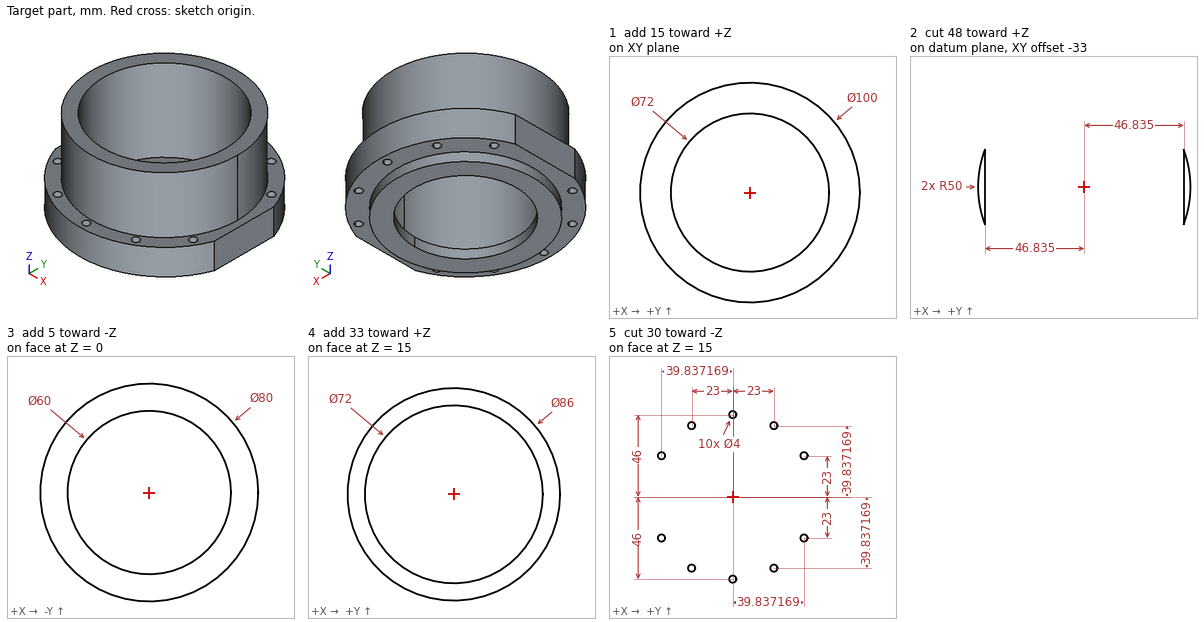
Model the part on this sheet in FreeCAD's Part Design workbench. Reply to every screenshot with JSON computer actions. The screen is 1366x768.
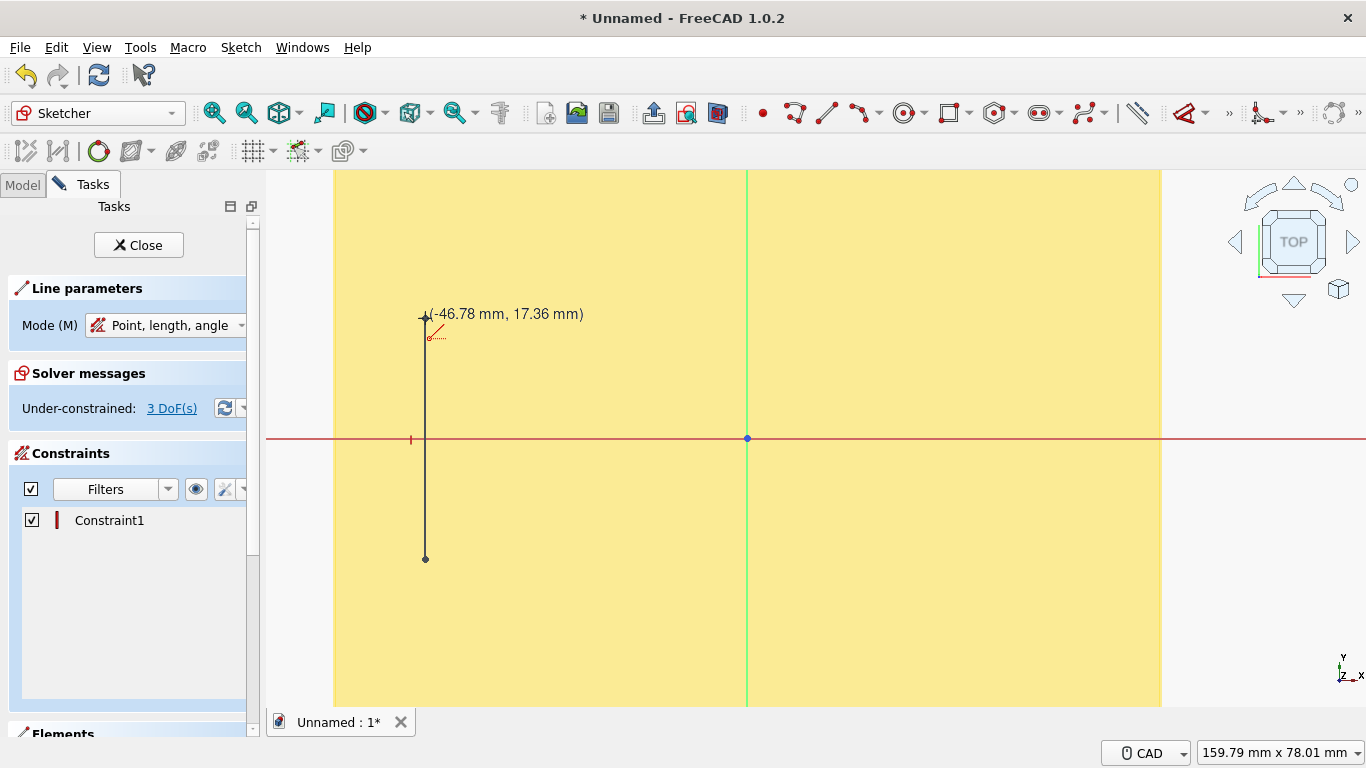
{"action": "left_click", "coordinate": [860, 114]}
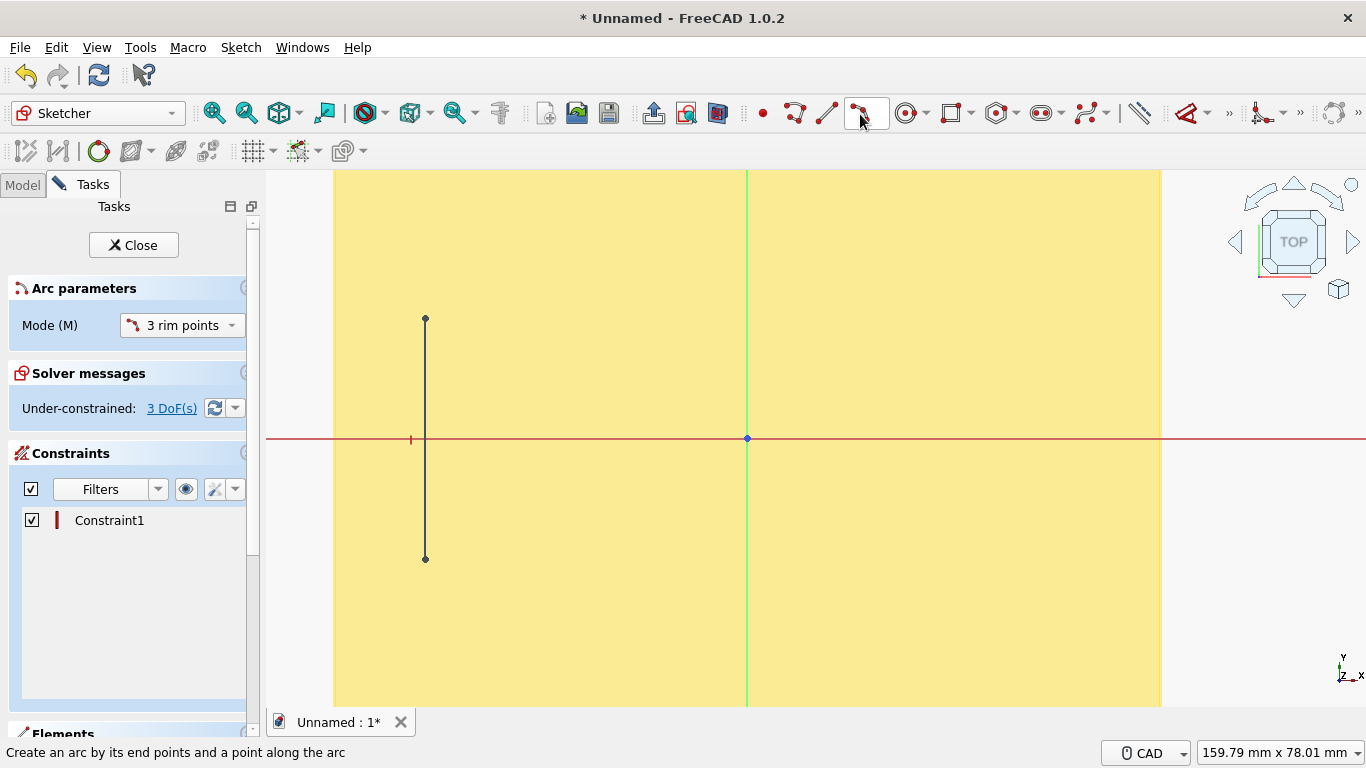
{"action": "left_click", "coordinate": [425, 319]}
{"action": "left_click", "coordinate": [425, 560]}
{"action": "left_click", "coordinate": [404, 414]}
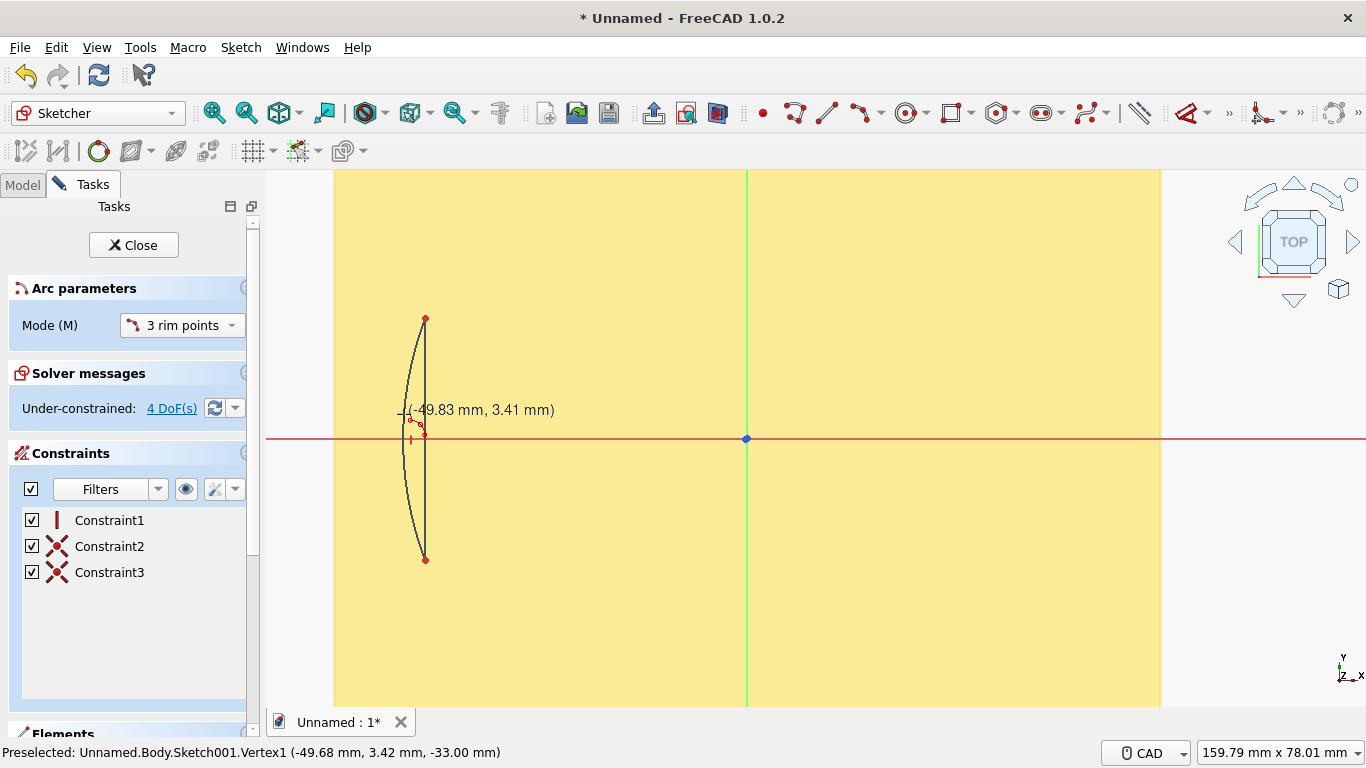
{"action": "left_click", "coordinate": [828, 114]}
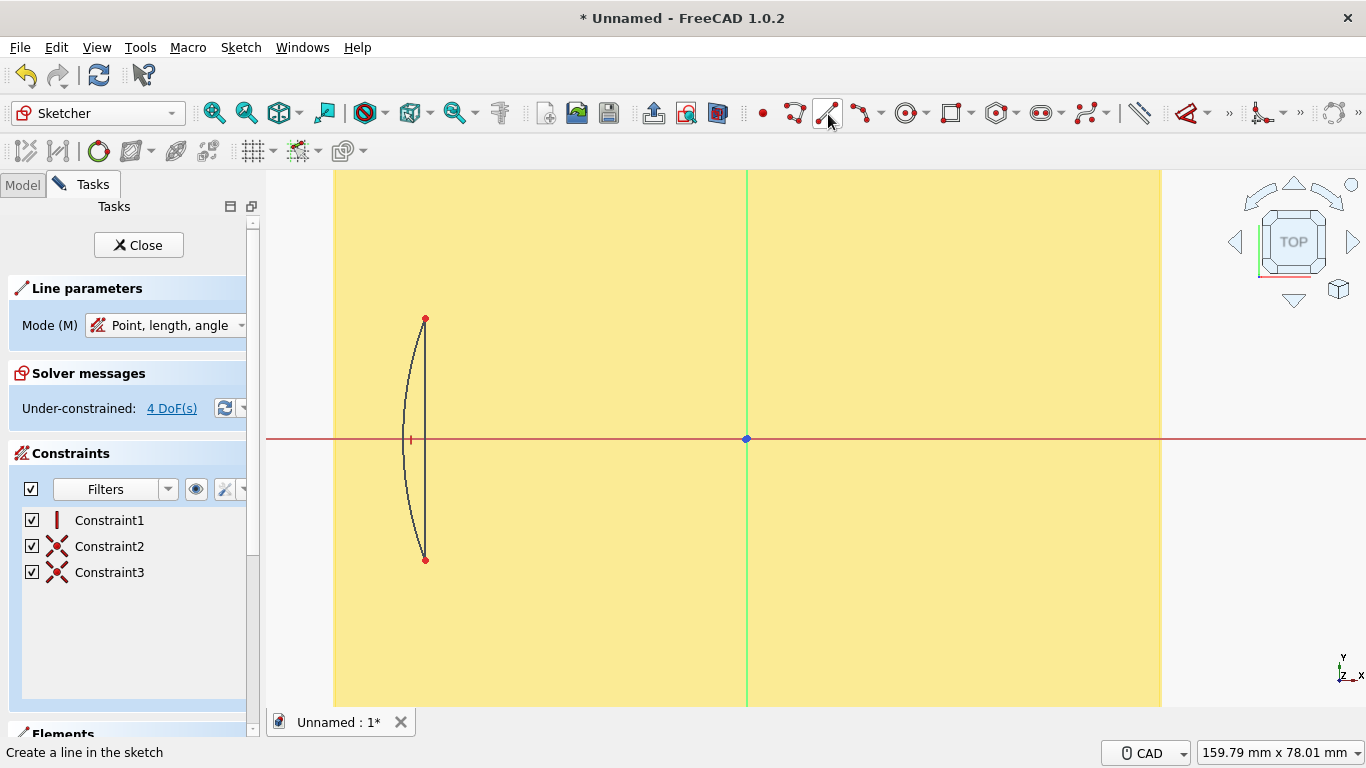
{"action": "left_click", "coordinate": [1069, 318]}
{"action": "left_click", "coordinate": [1069, 559]}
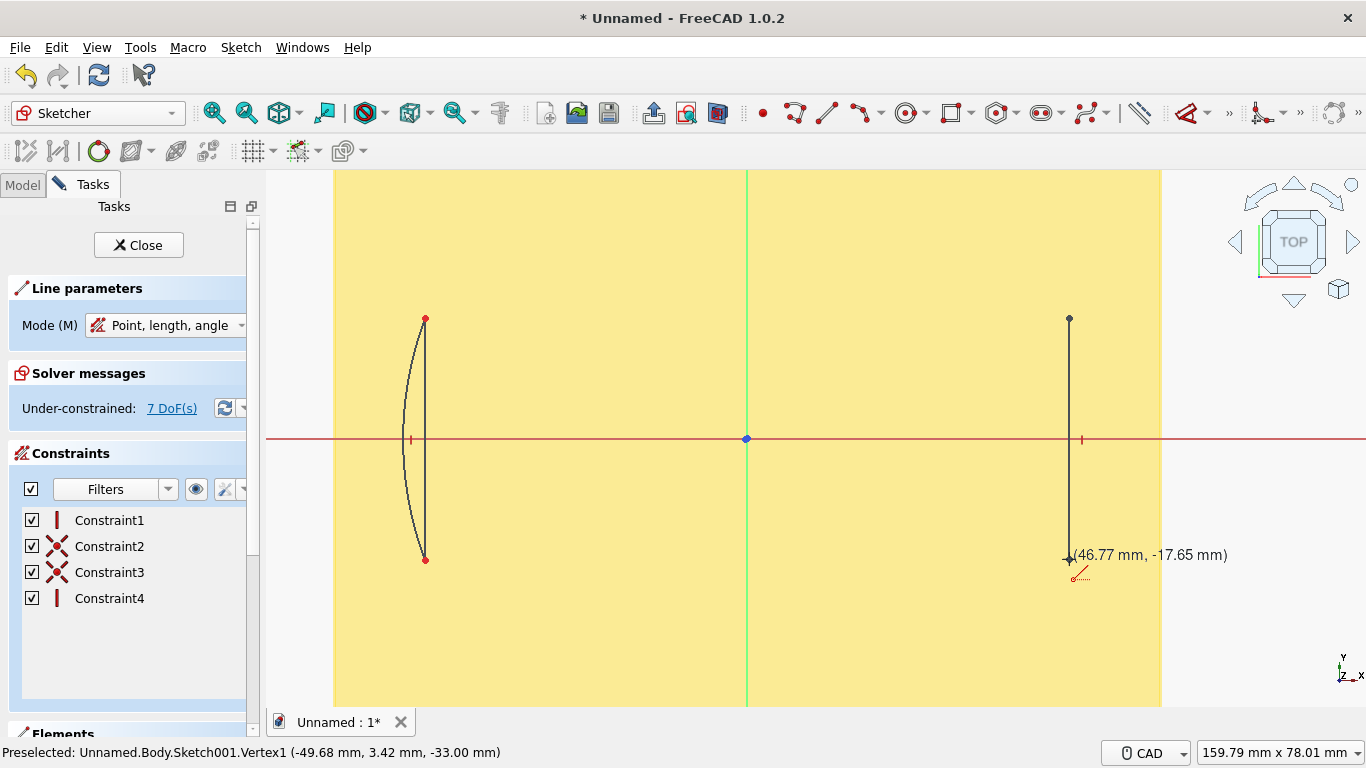
{"action": "left_click", "coordinate": [860, 114]}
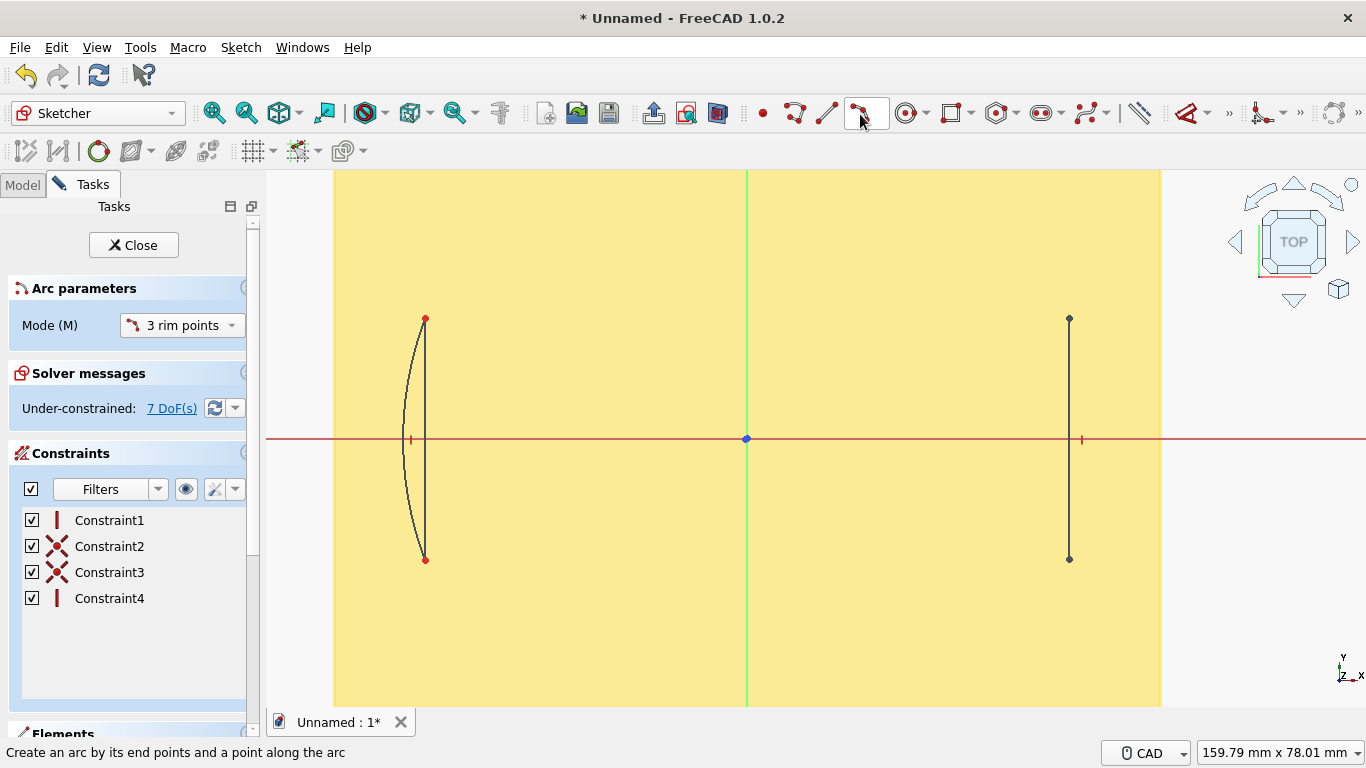
{"action": "left_click", "coordinate": [1069, 560]}
{"action": "left_click", "coordinate": [1069, 319]}
{"action": "left_click", "coordinate": [1090, 463]}
{"action": "key", "text": "Escape"}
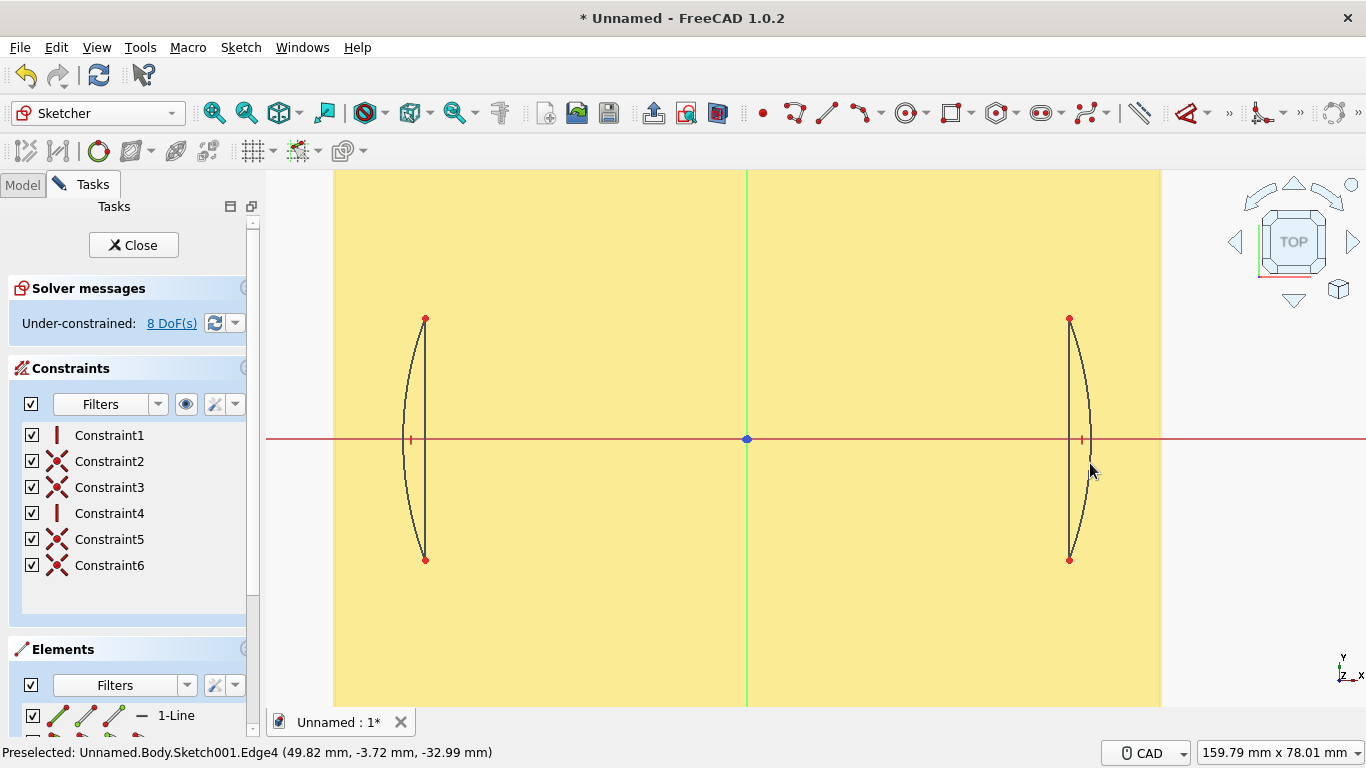
{"action": "left_click", "coordinate": [407, 390]}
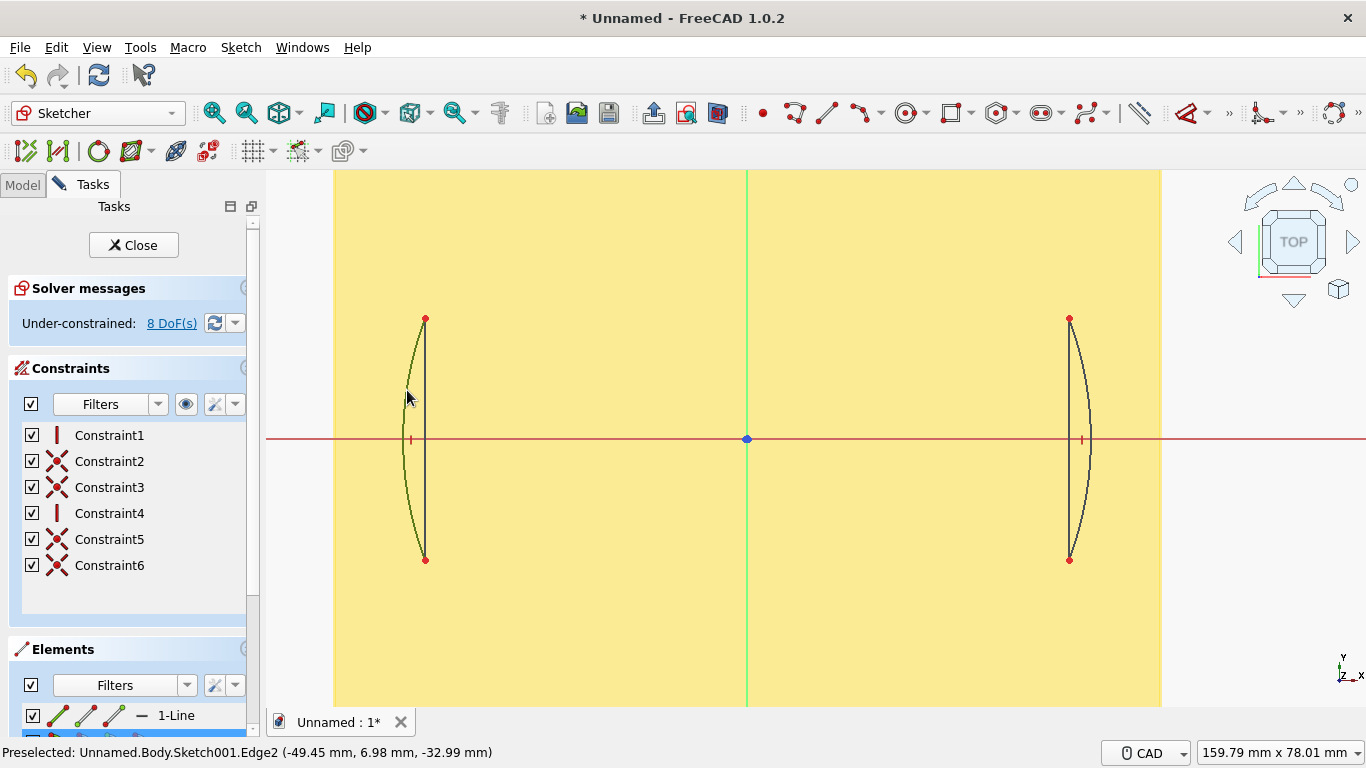
{"action": "left_click", "coordinate": [1087, 489]}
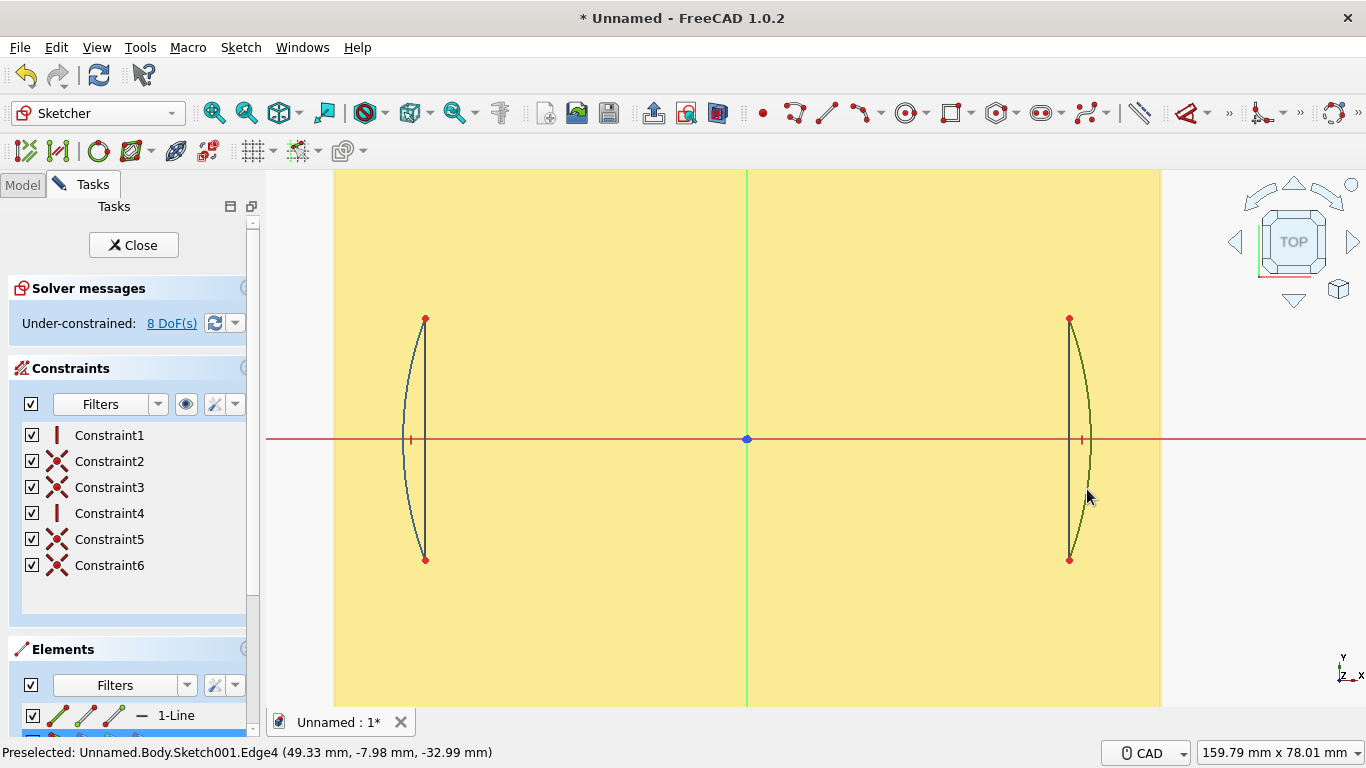
{"action": "key", "text": "c"}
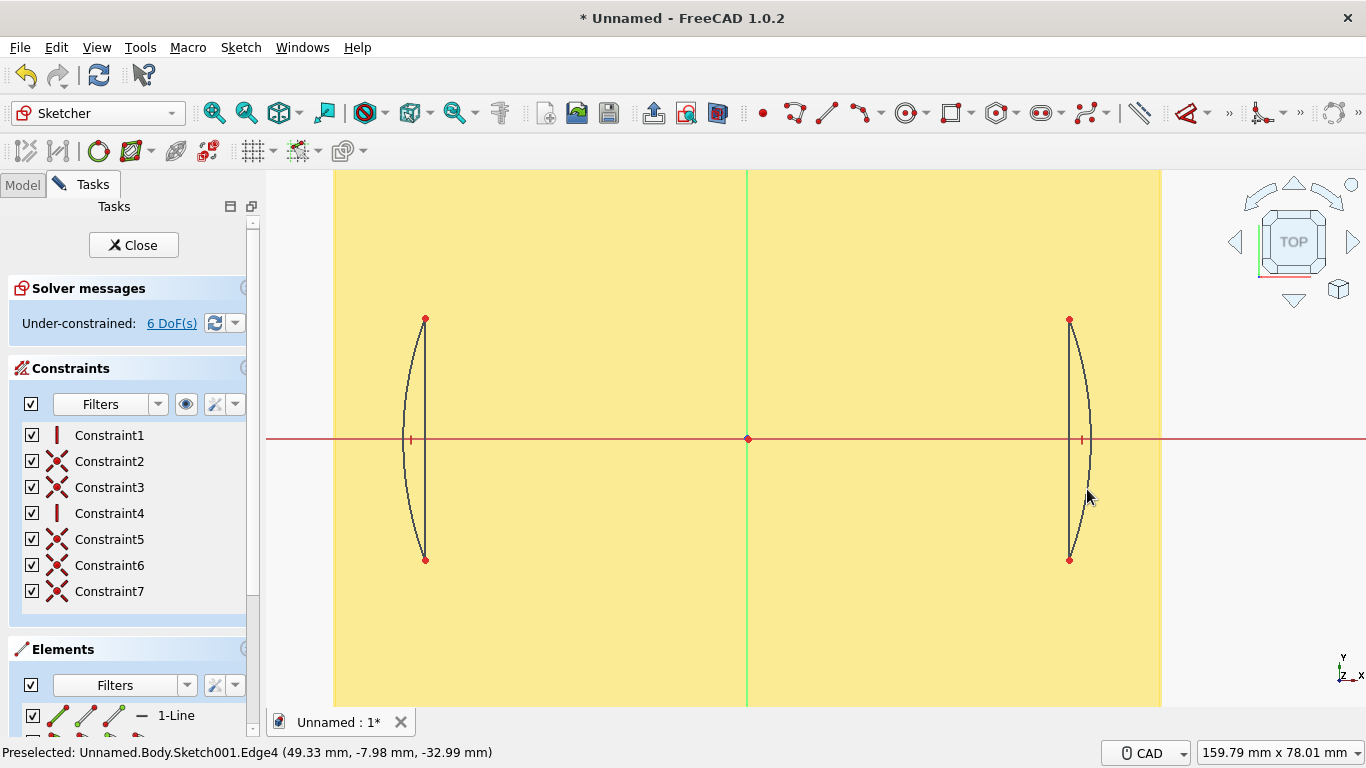
{"action": "left_click_drag", "start_coordinate": [737, 428], "coordinate": [758, 450]}